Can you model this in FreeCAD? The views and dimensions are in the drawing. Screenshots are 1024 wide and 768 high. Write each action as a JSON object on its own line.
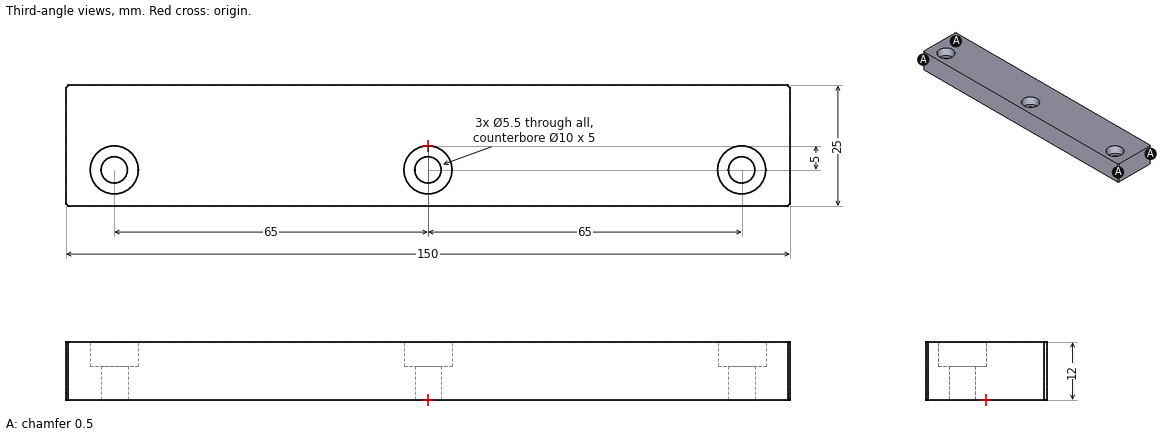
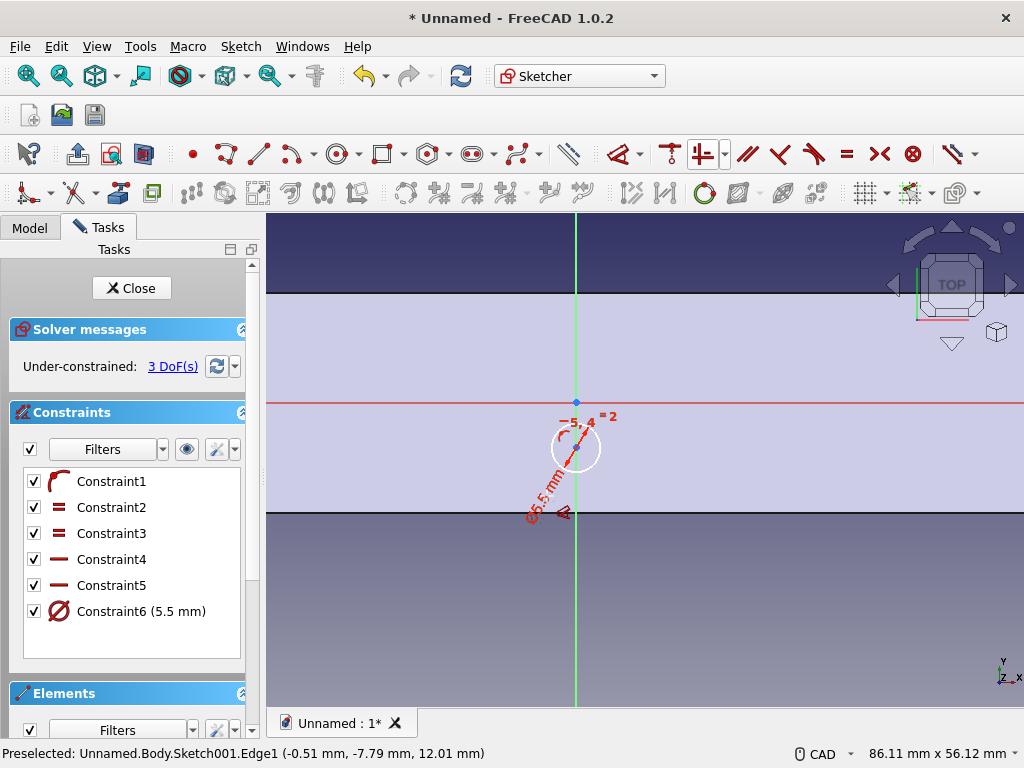
{"action": "left_click", "coordinate": [576, 448]}
{"action": "left_click", "coordinate": [610, 425]}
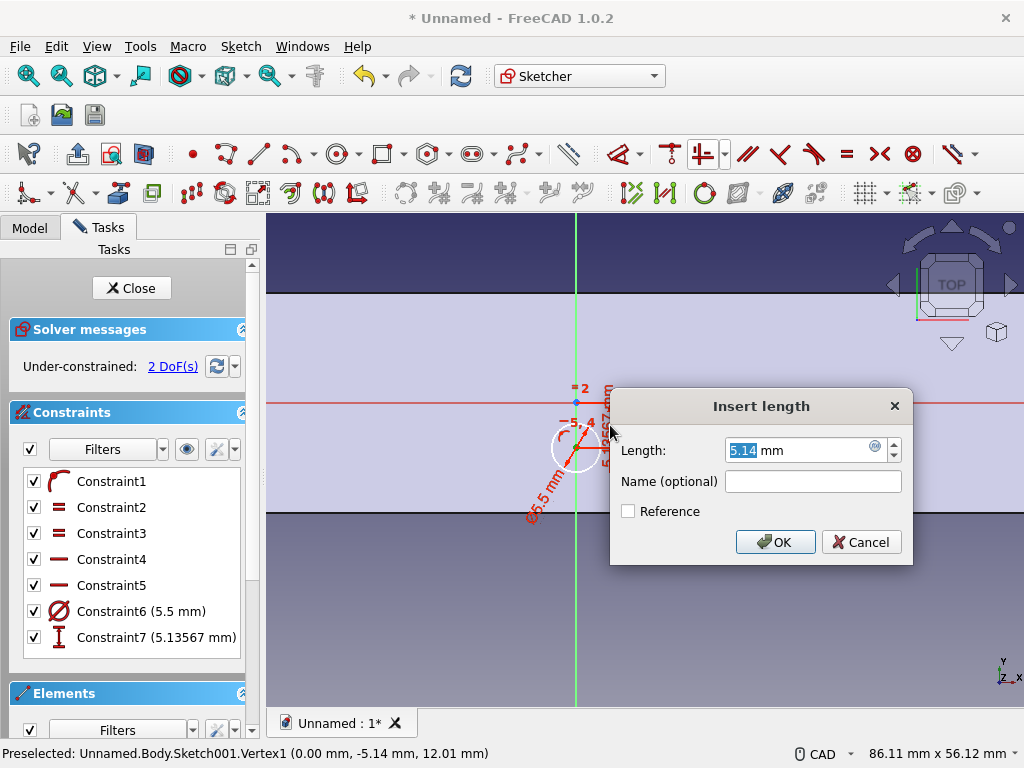
{"action": "type", "text": "5"}
{"action": "key", "text": "Return"}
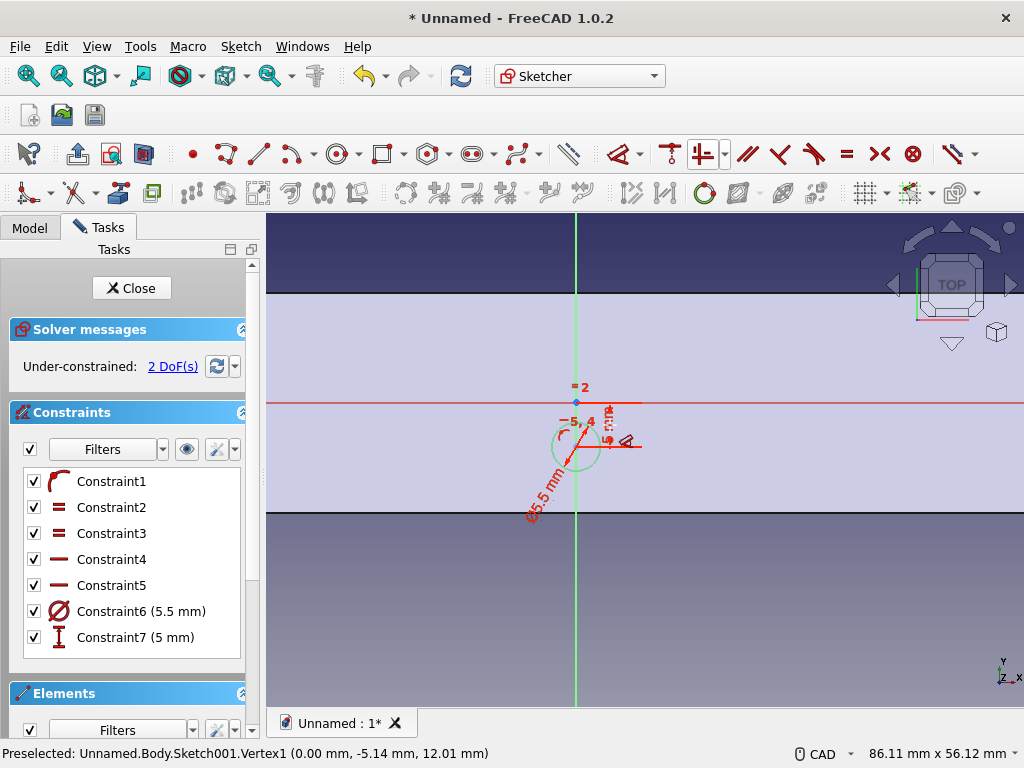
{"action": "scroll", "coordinate": [577, 473], "scroll_direction": "down", "scroll_amount": 5}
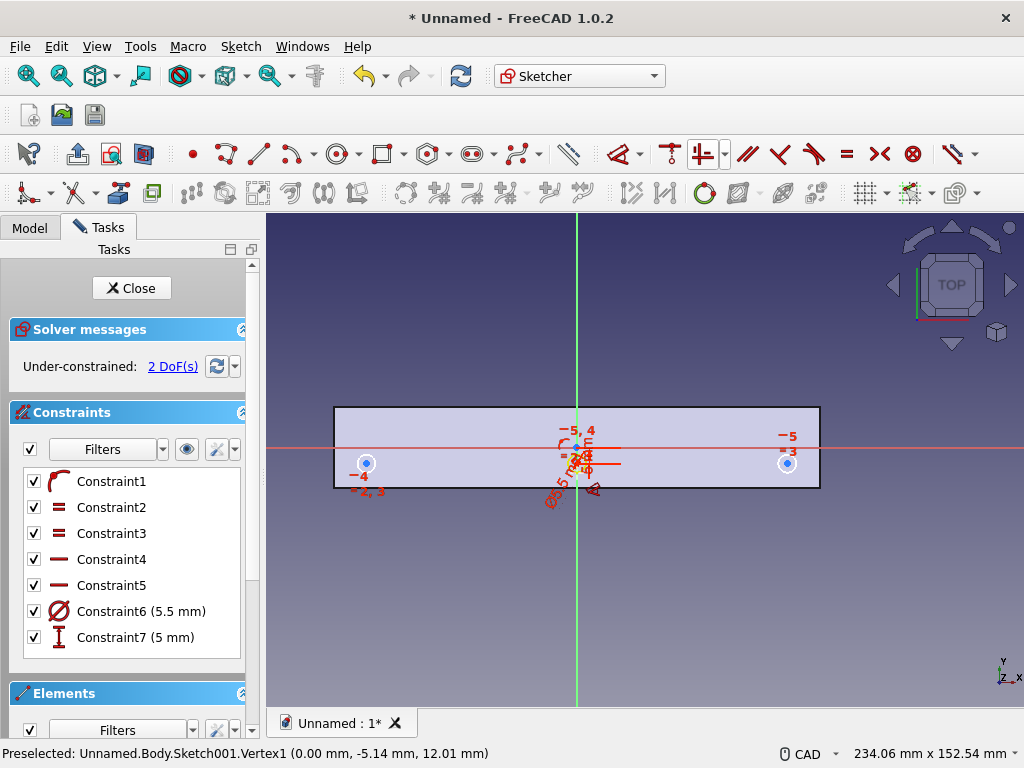
{"action": "left_click", "coordinate": [366, 464]}
{"action": "left_click", "coordinate": [472, 414]}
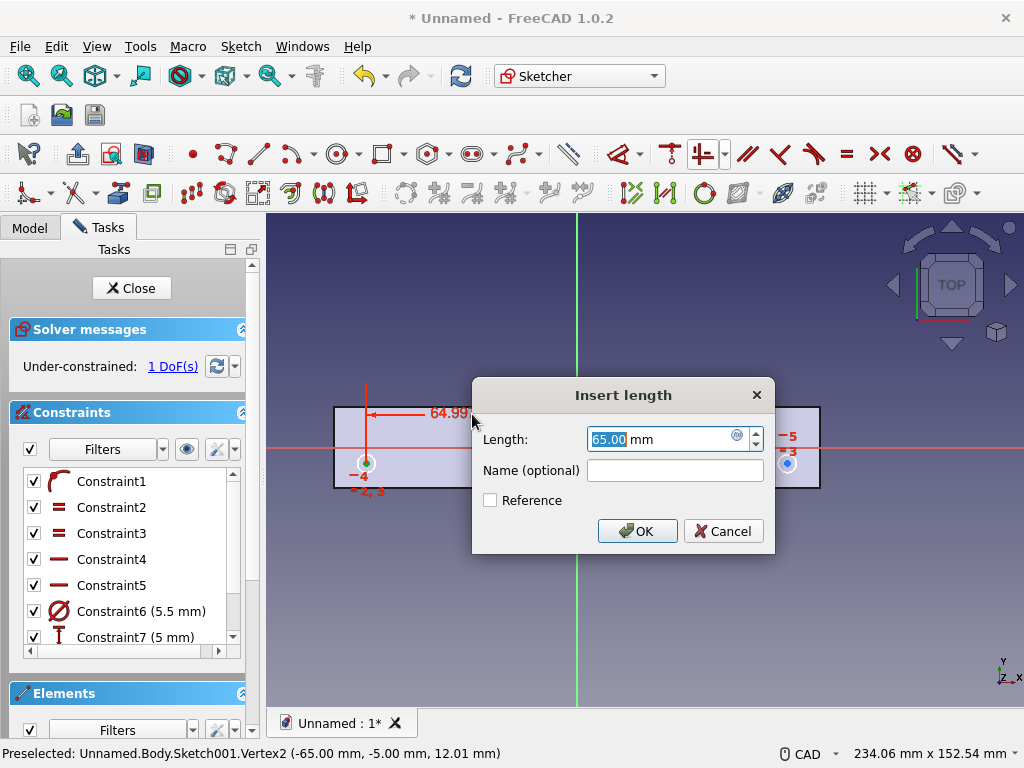
{"action": "type", "text": "65"}
{"action": "key", "text": "Return"}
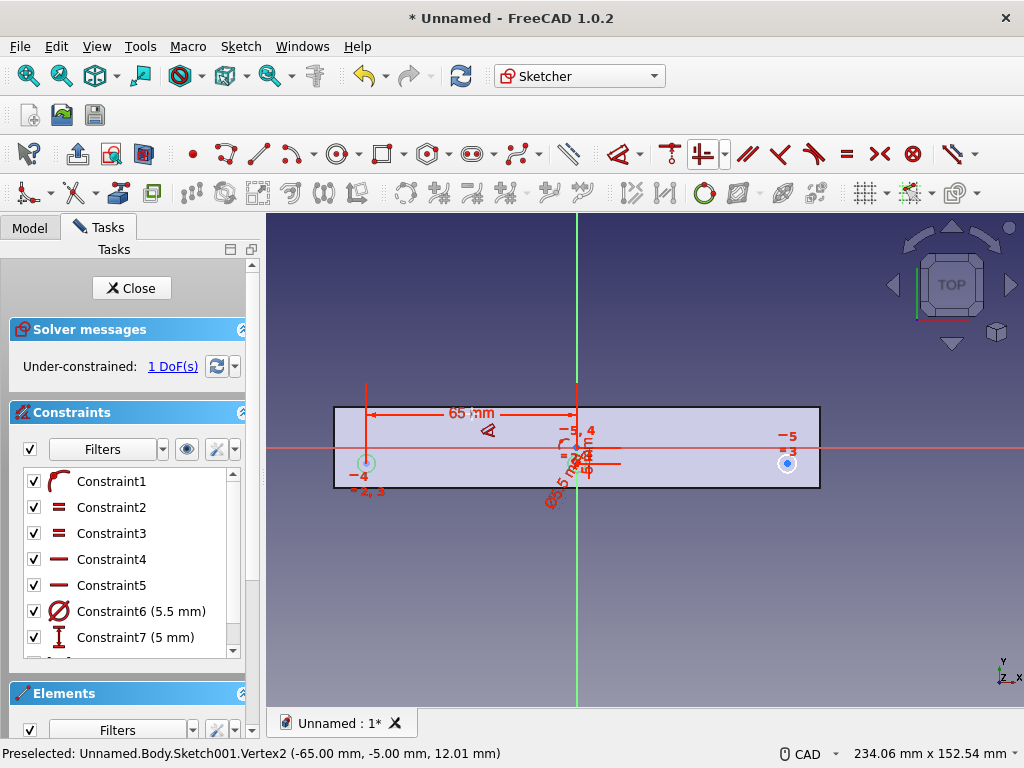
{"action": "left_click", "coordinate": [787, 464]}
{"action": "left_click", "coordinate": [682, 414]}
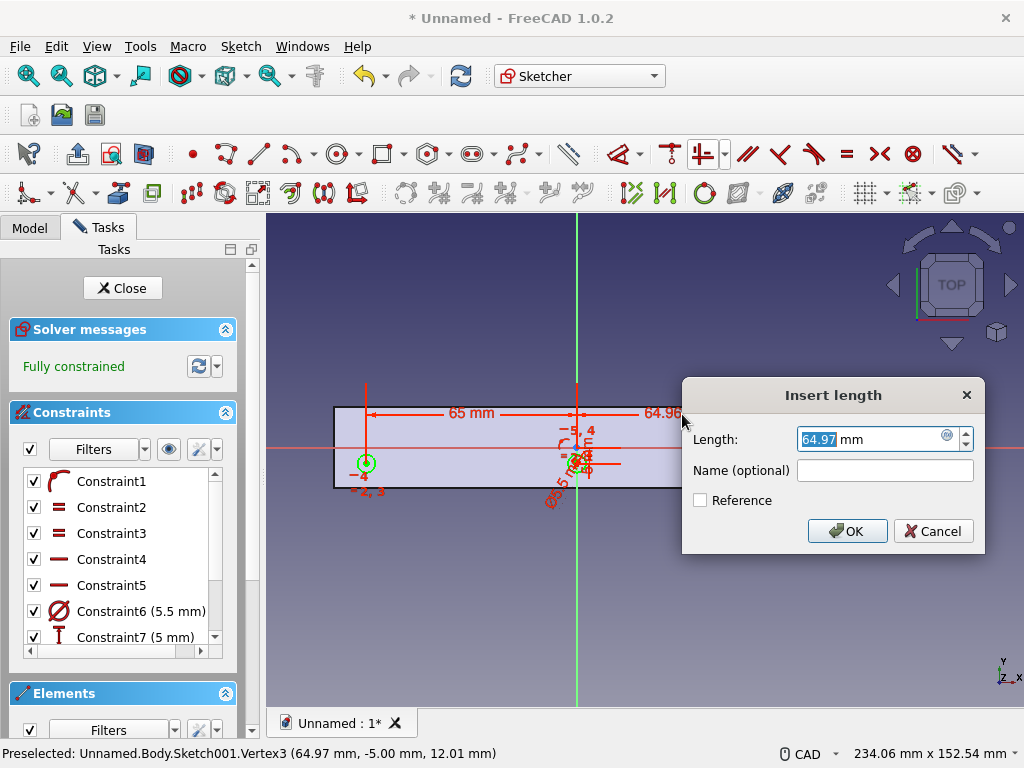
{"action": "type", "text": "65"}
{"action": "key", "text": "Return"}
{"action": "key", "text": "Escape"}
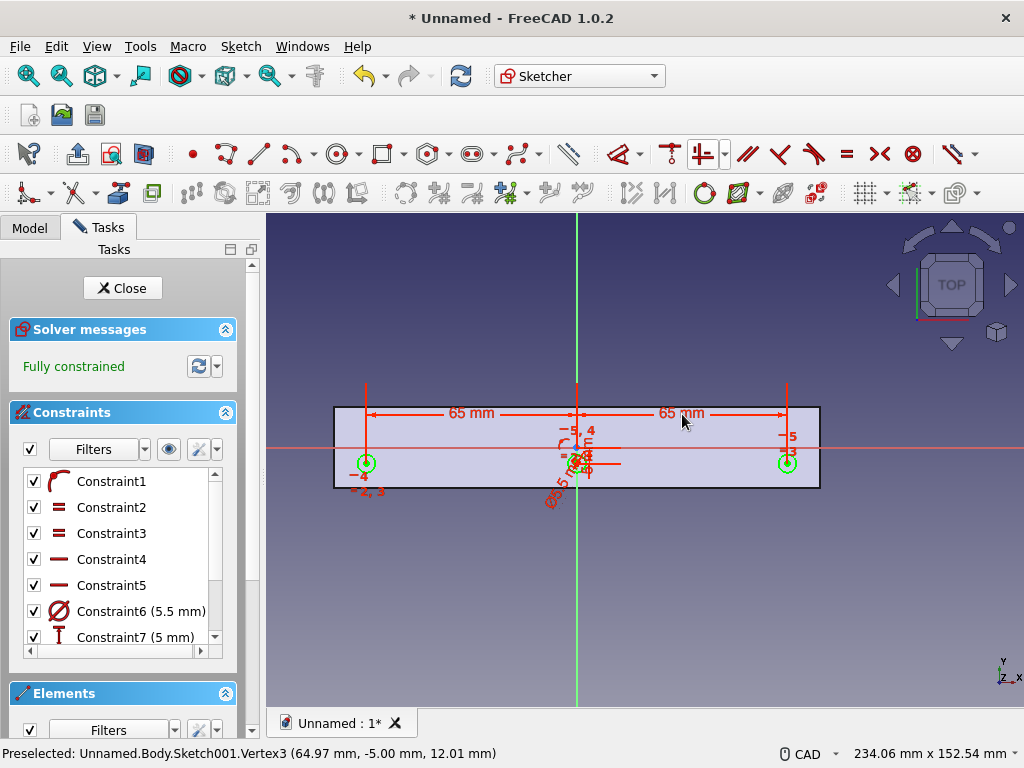
{"action": "left_click", "coordinate": [123, 288]}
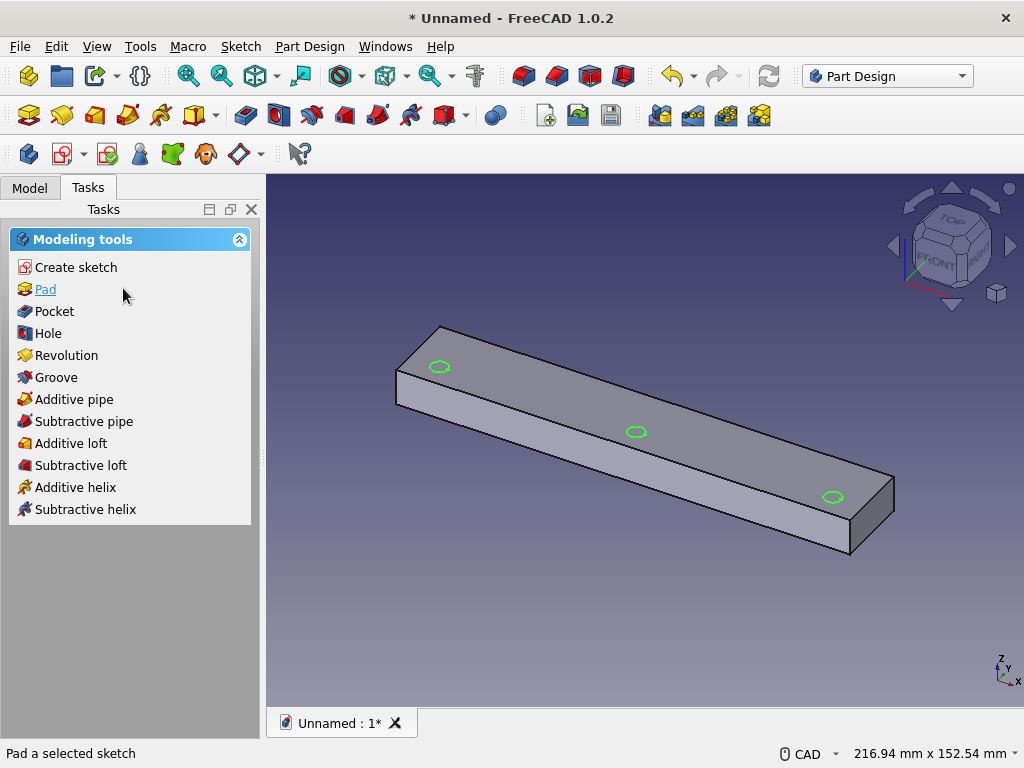
{"action": "left_click", "coordinate": [279, 116]}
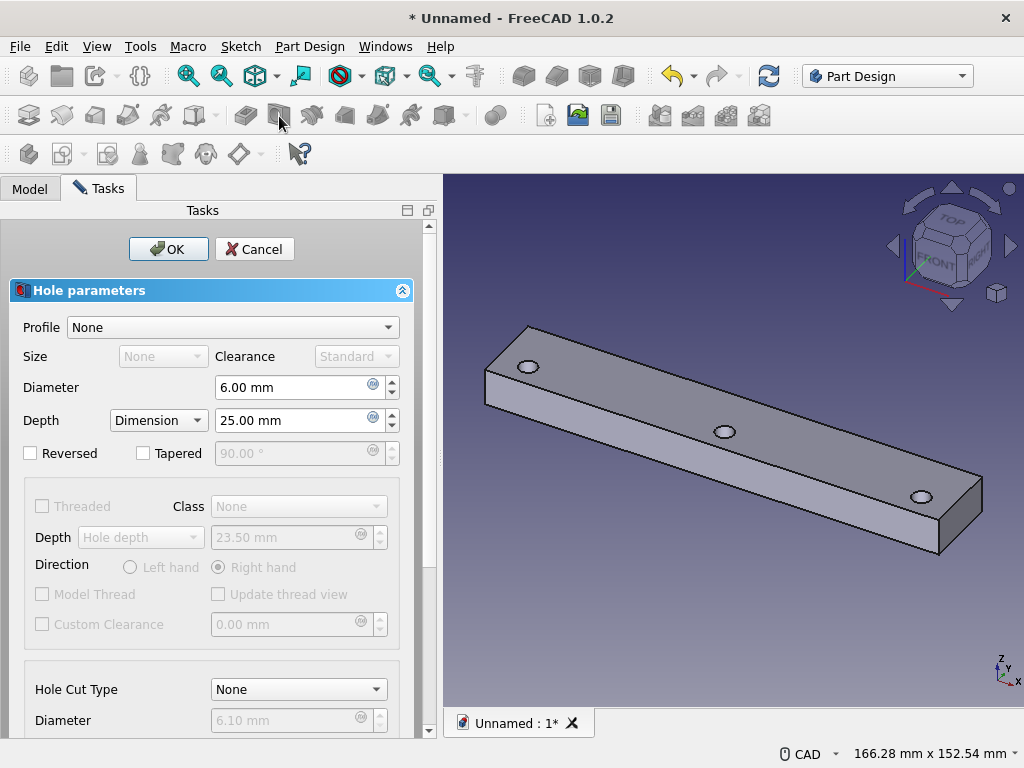
{"action": "triple_click", "coordinate": [300, 388]}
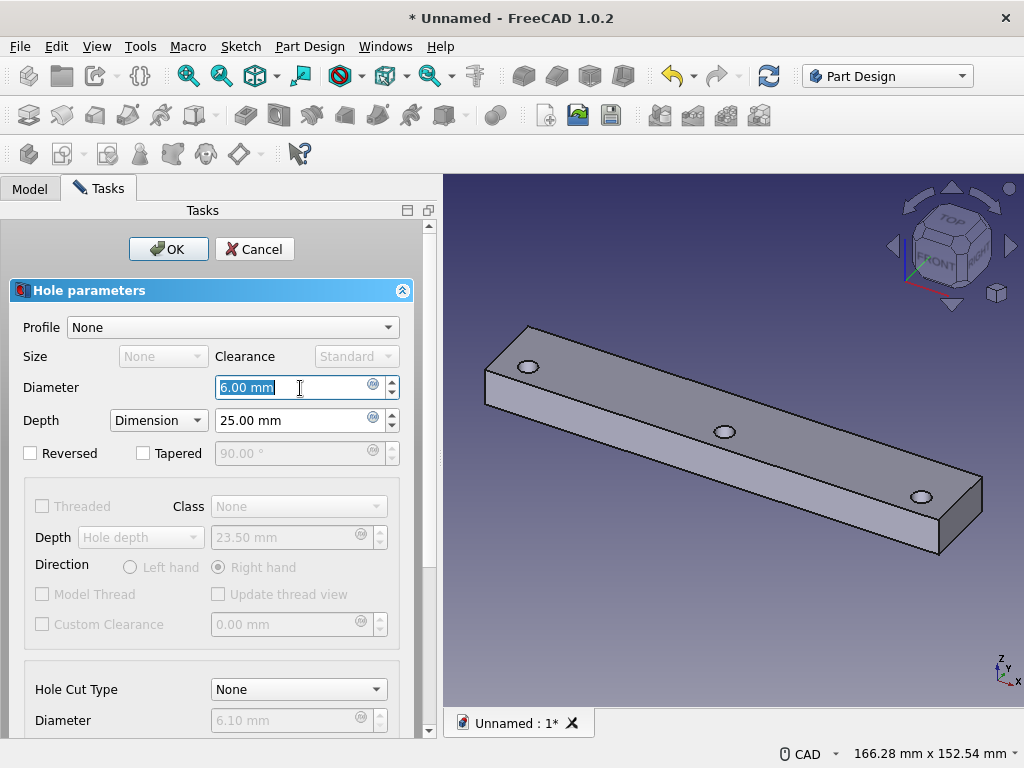
{"action": "type", "text": "5.5"}
{"action": "key", "text": "Tab"}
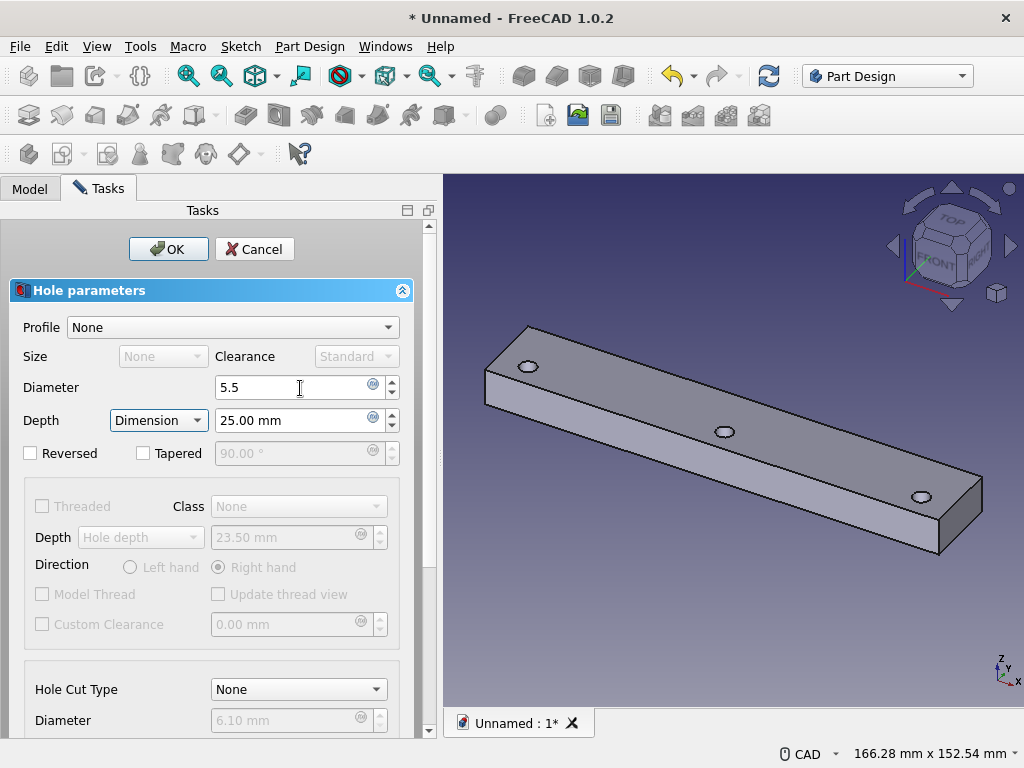
{"action": "left_click", "coordinate": [160, 420]}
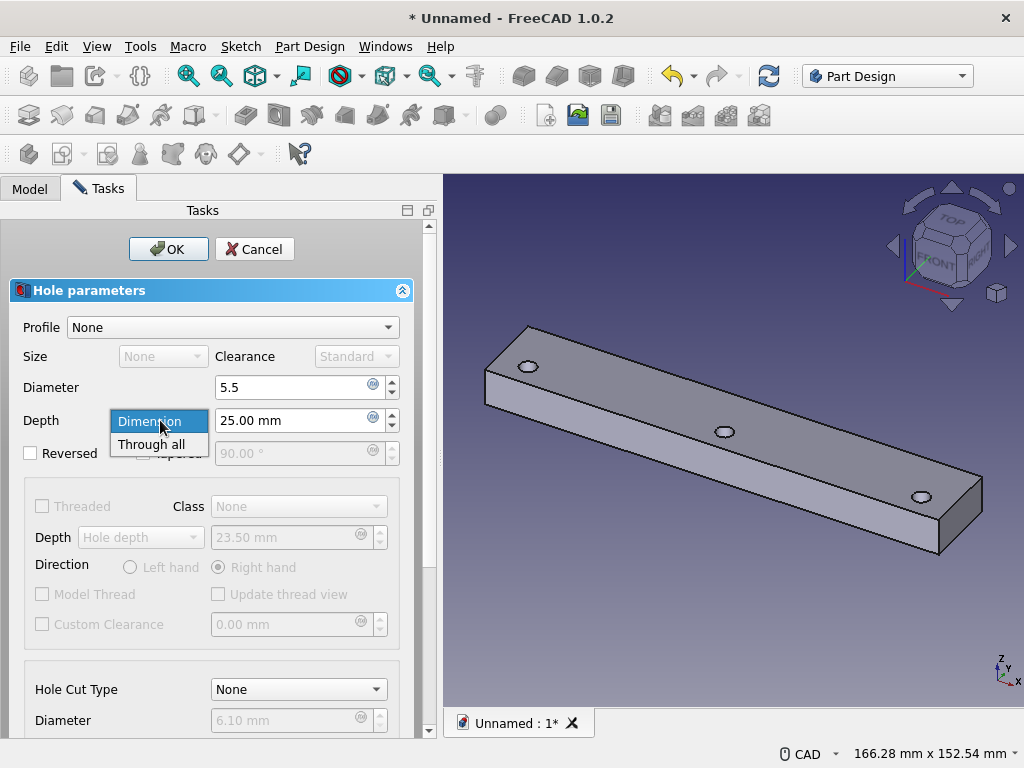
{"action": "left_click", "coordinate": [158, 444]}